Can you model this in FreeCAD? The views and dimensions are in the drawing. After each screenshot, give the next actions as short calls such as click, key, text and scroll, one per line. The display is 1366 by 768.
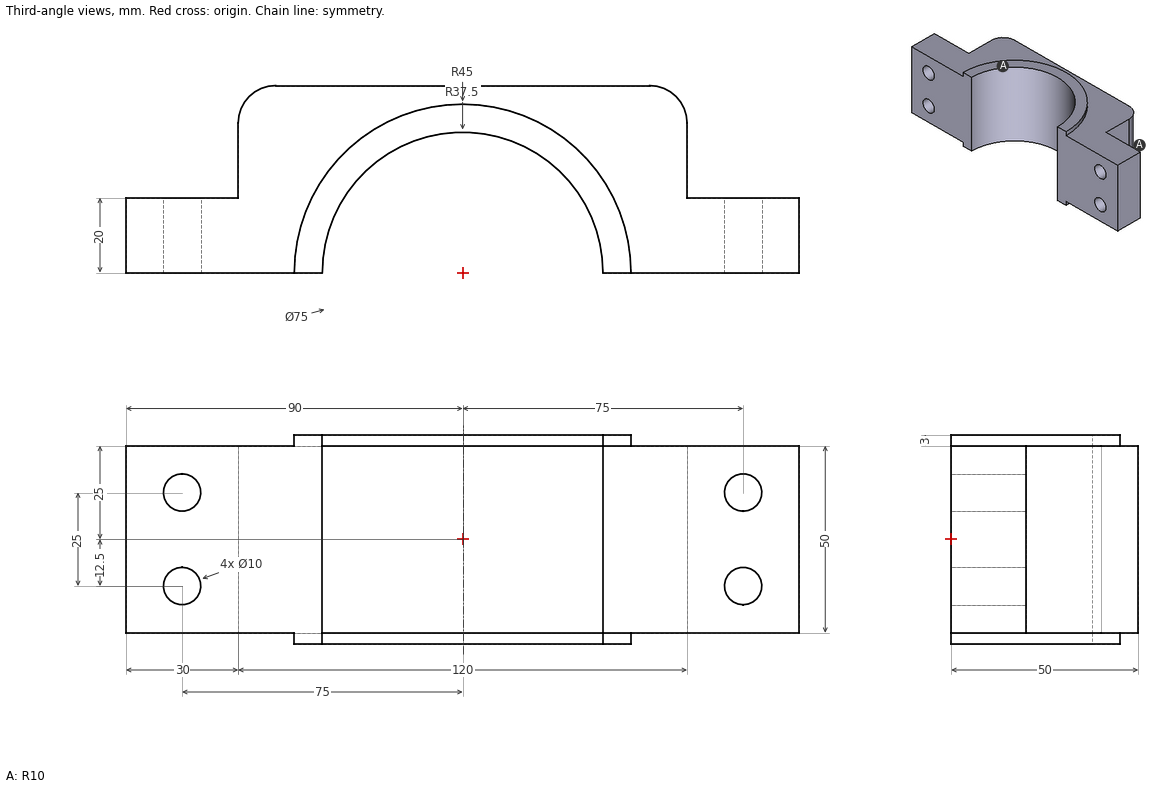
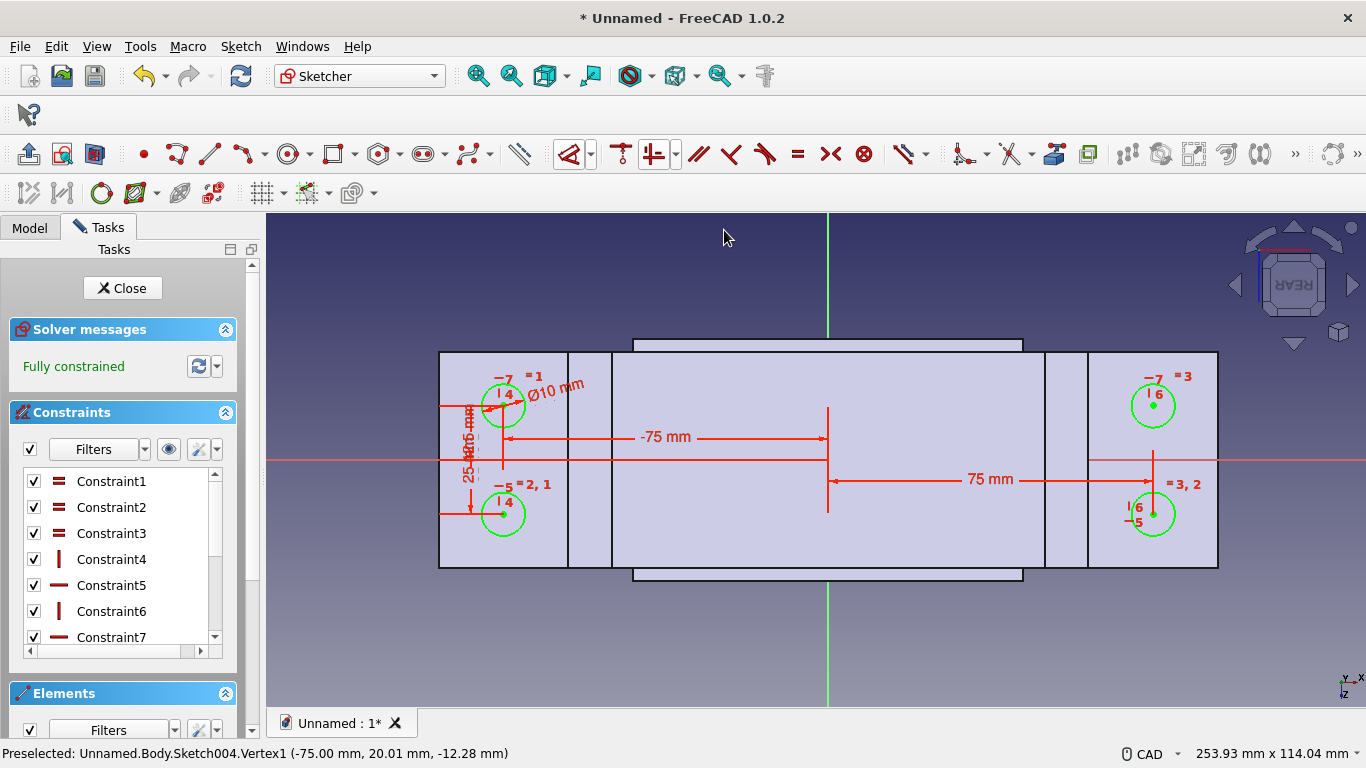
click(123, 288)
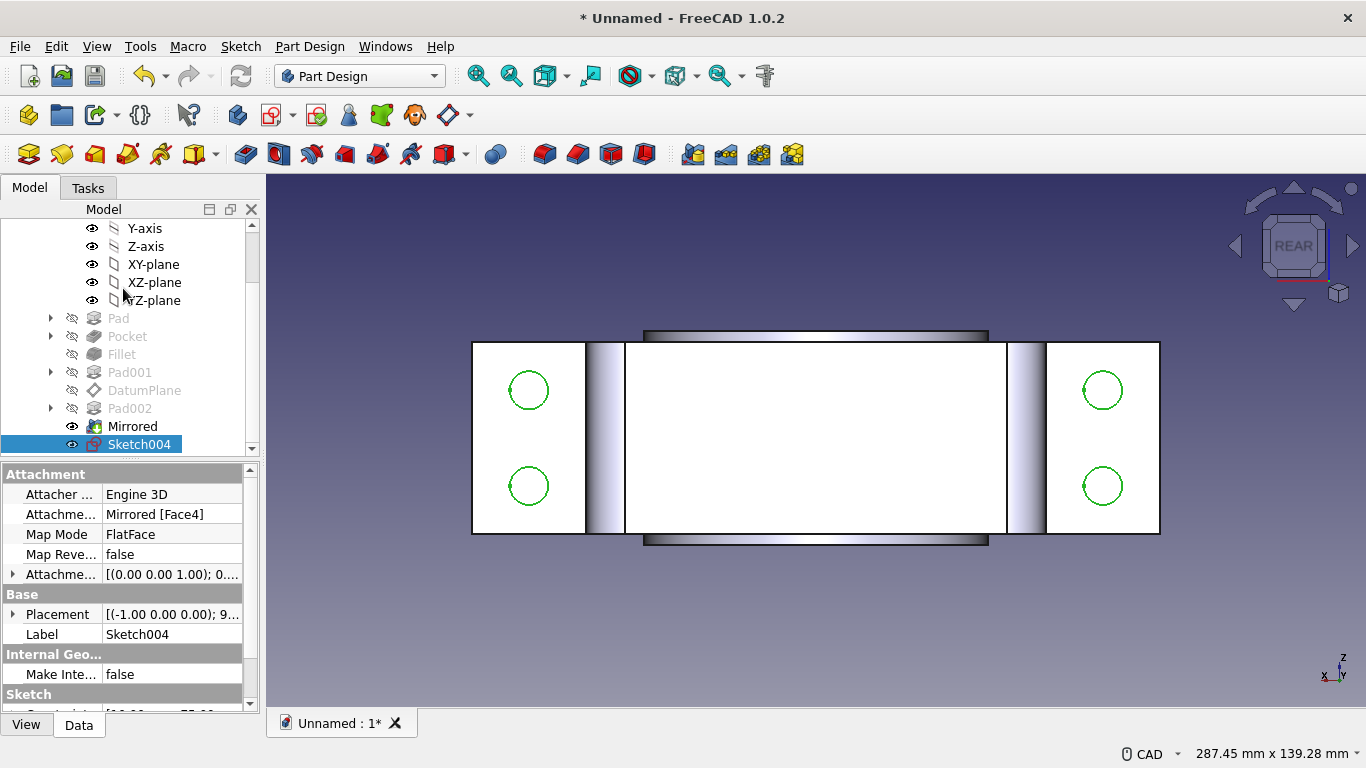
click(246, 154)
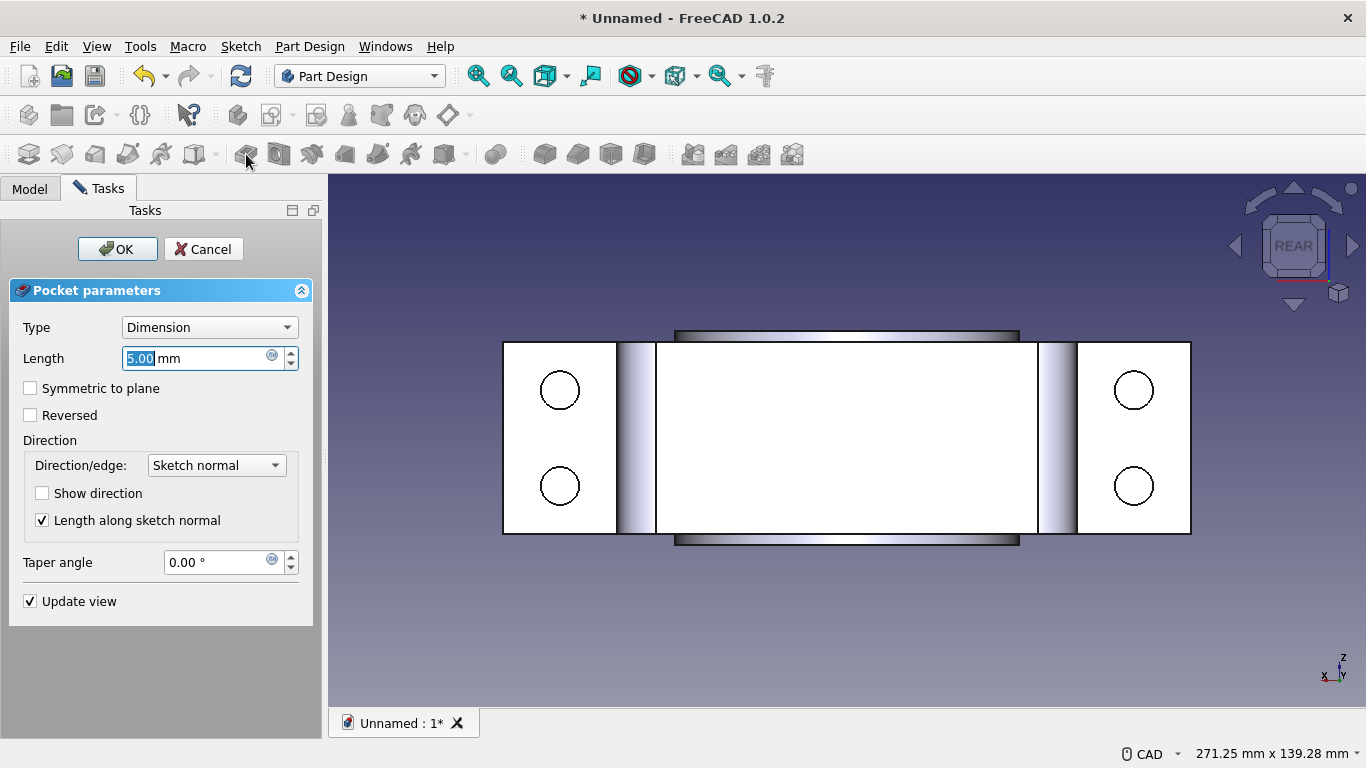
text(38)
key(Tab)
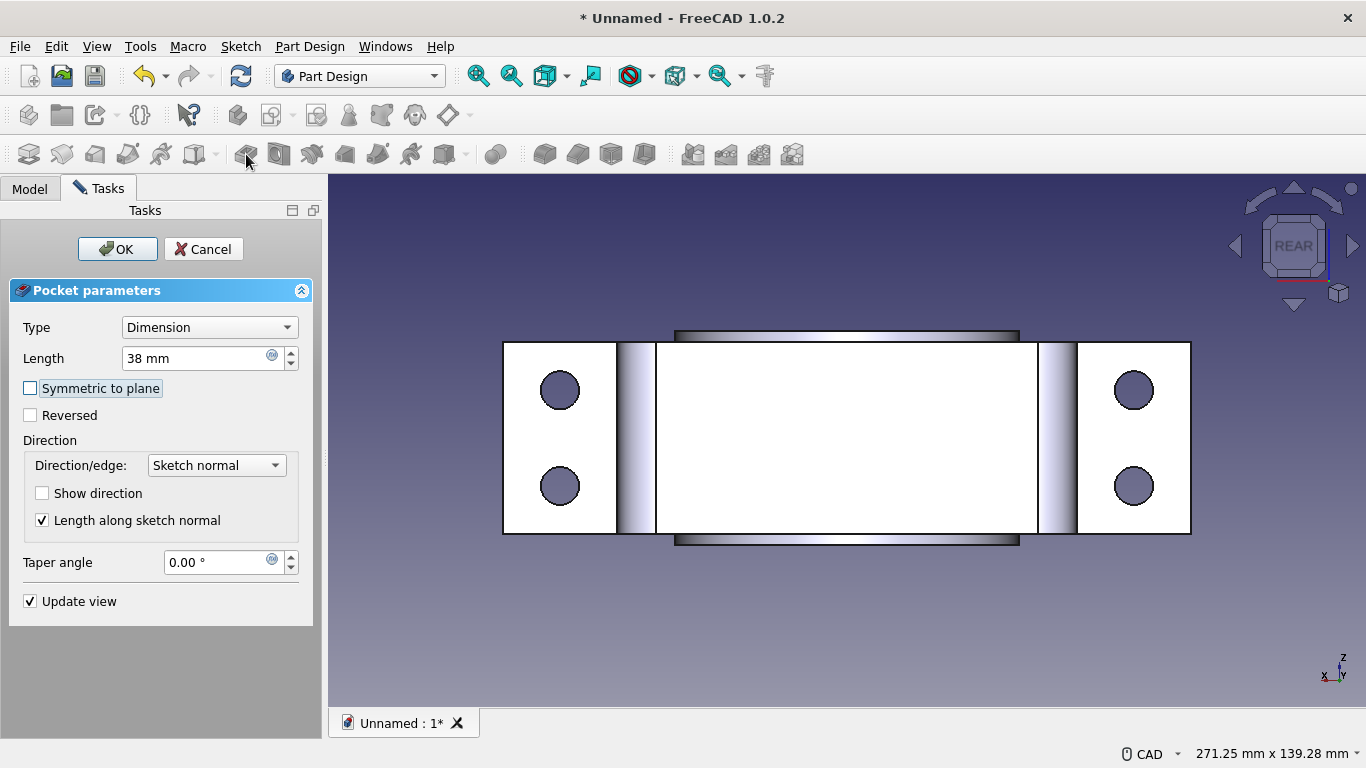
click(118, 249)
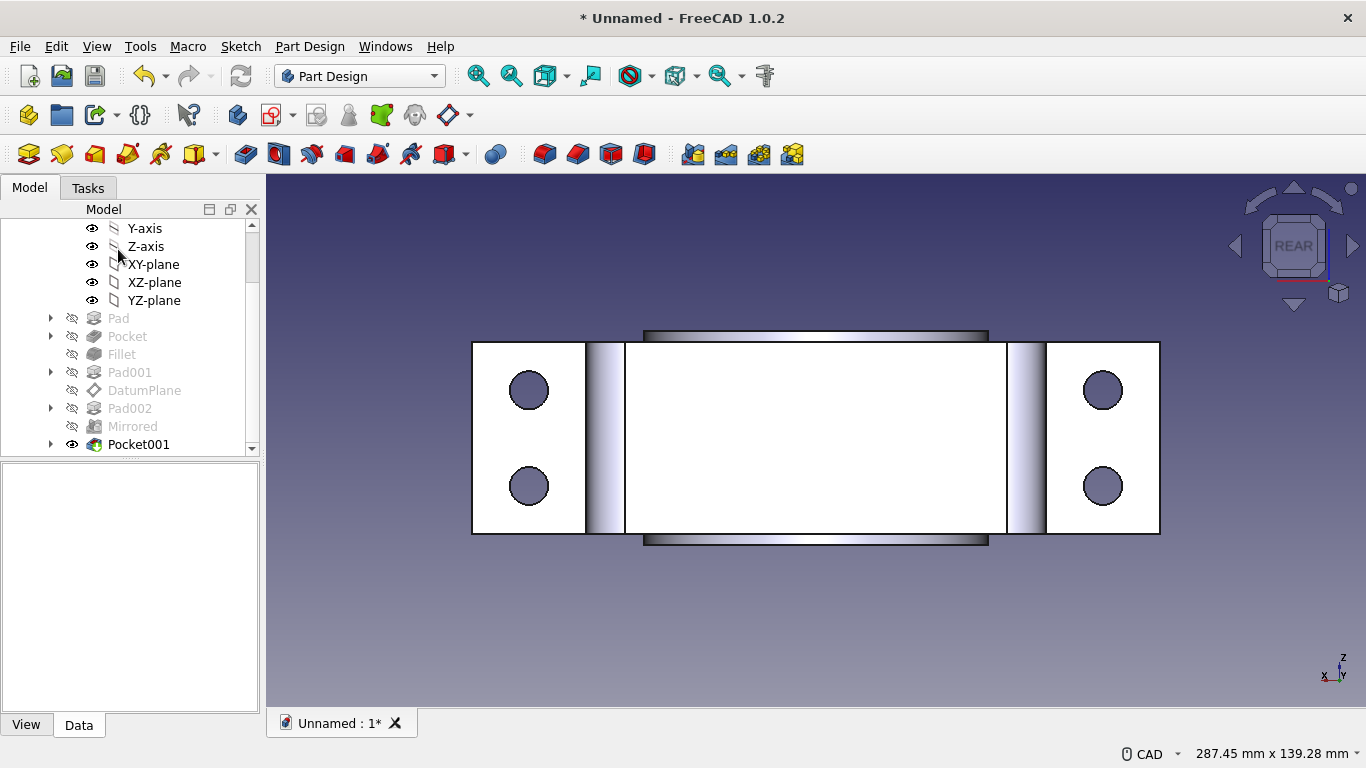
key(0)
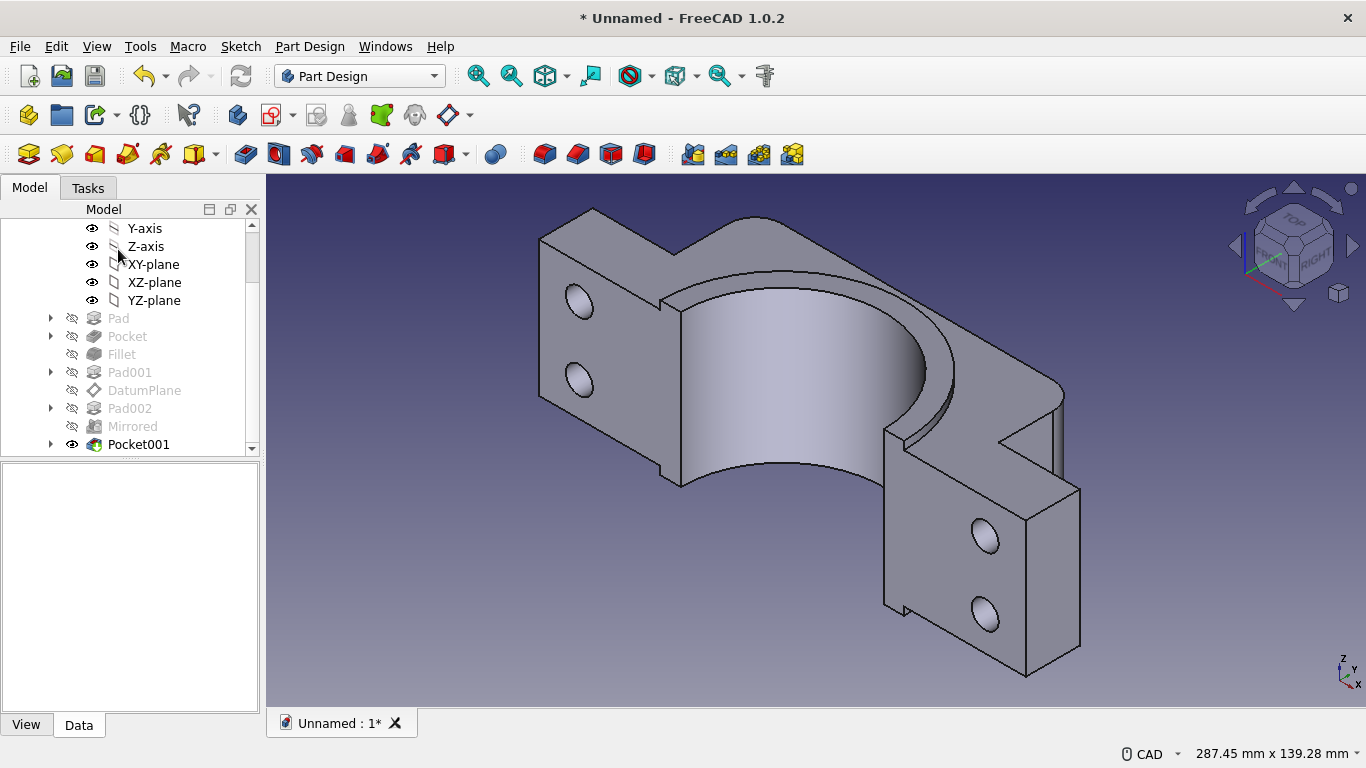
click(479, 76)